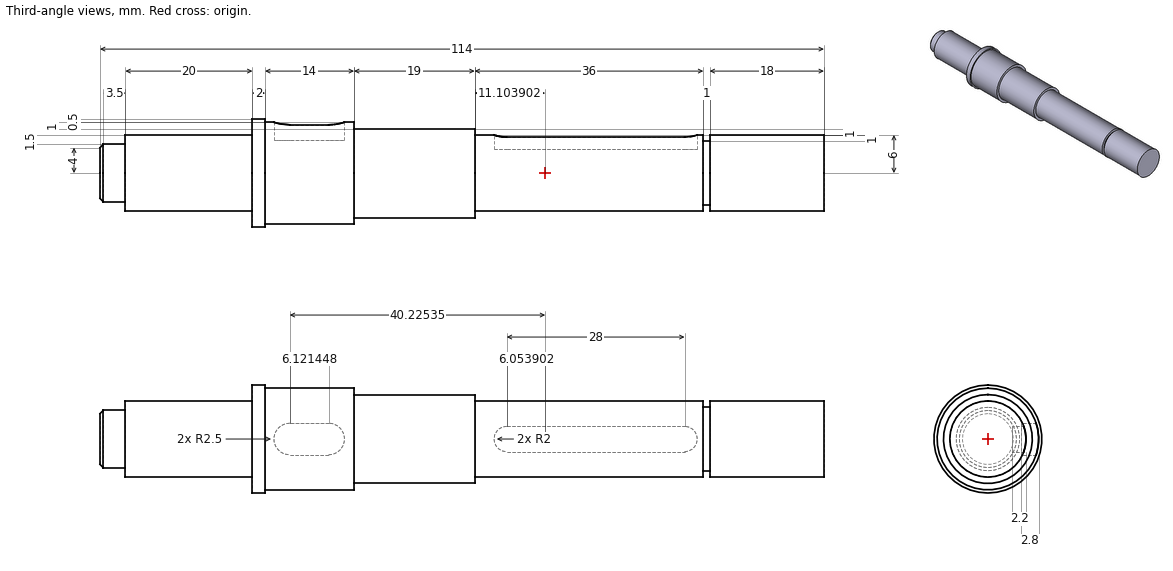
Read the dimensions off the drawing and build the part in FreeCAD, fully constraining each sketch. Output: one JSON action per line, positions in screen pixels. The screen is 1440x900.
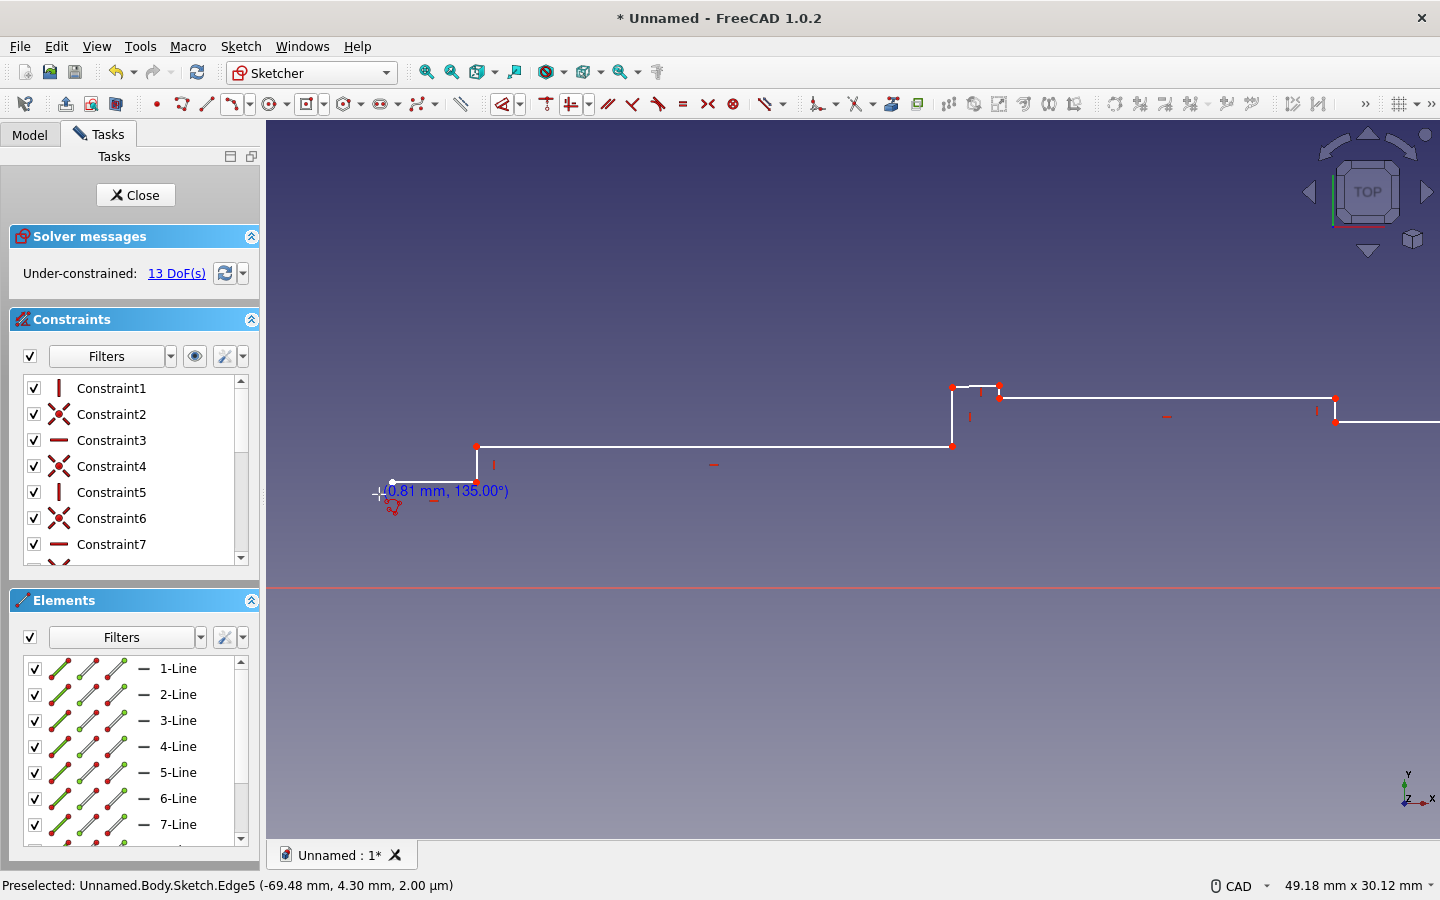
{"action": "left_click", "coordinate": [380, 492]}
{"action": "left_click", "coordinate": [380, 588]}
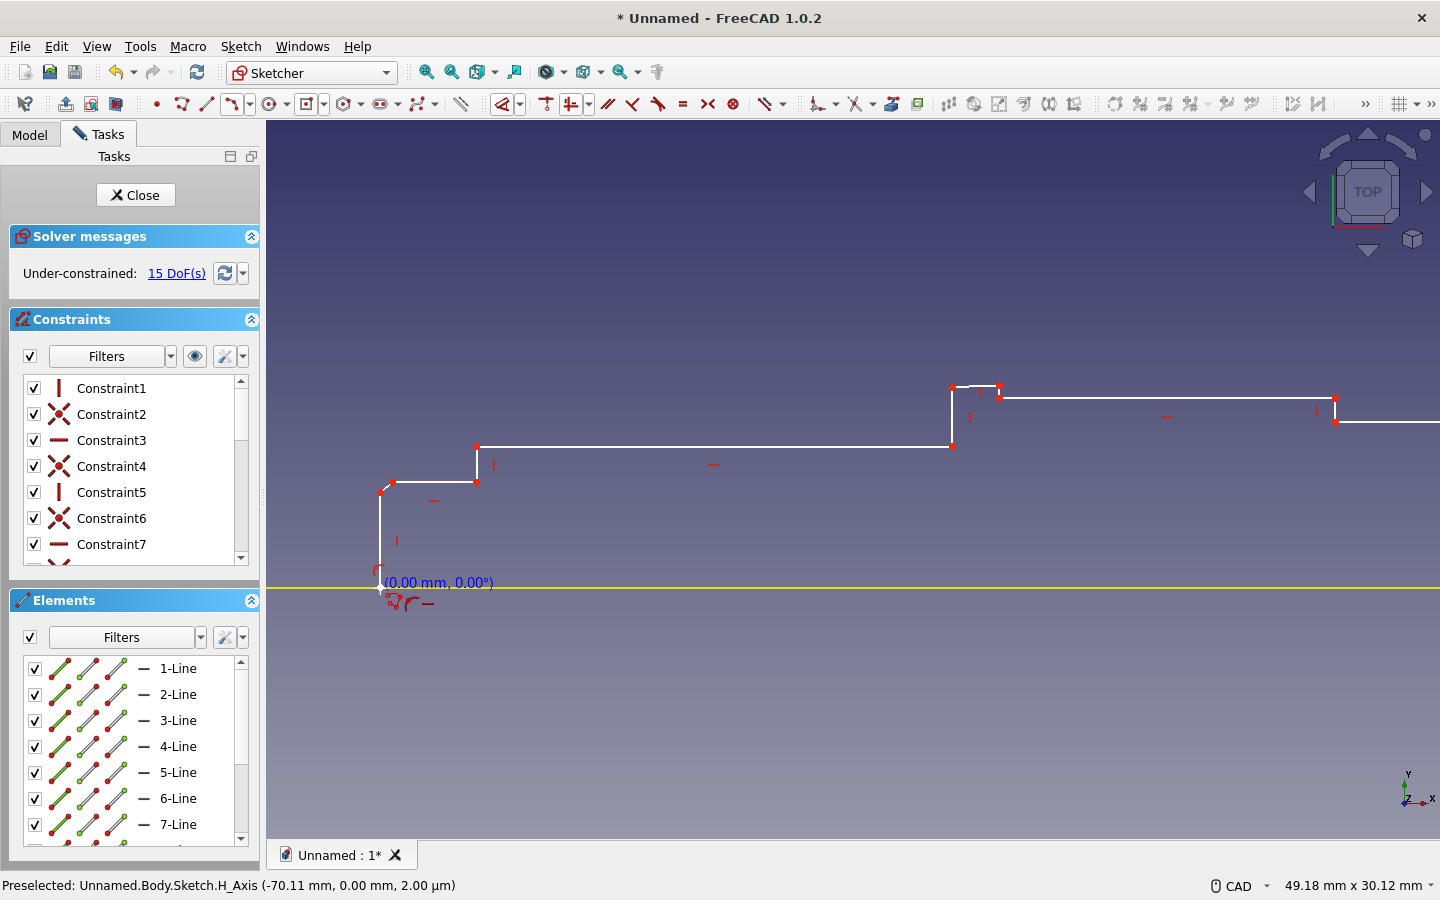
{"action": "scroll", "coordinate": [471, 477], "scroll_direction": "down", "scroll_amount": 7}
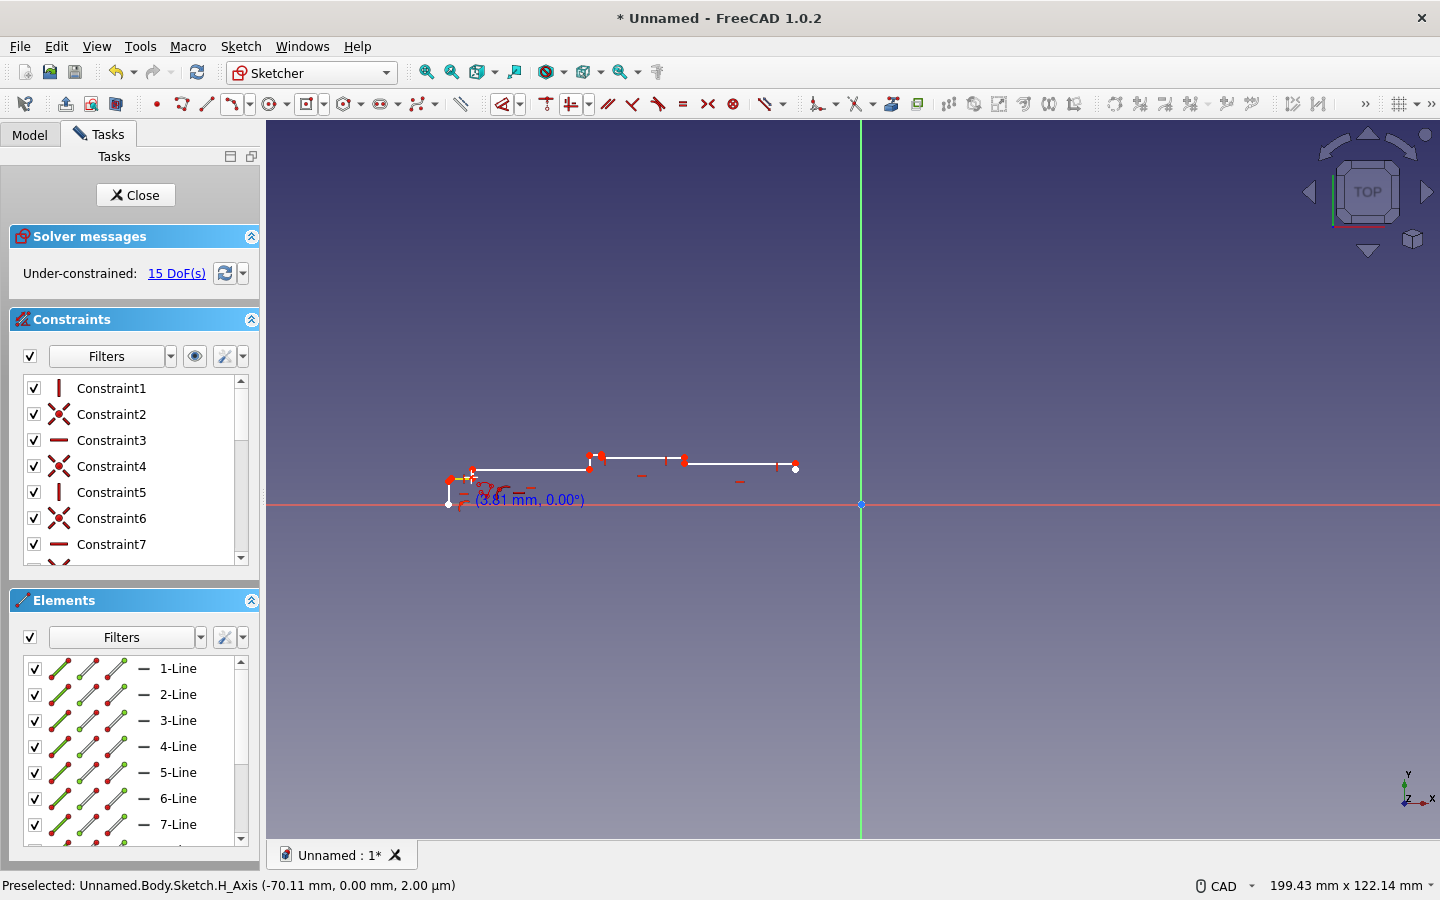
{"action": "left_click", "coordinate": [1120, 496]}
{"action": "left_click", "coordinate": [1120, 469]}
{"action": "left_click", "coordinate": [1014, 469]}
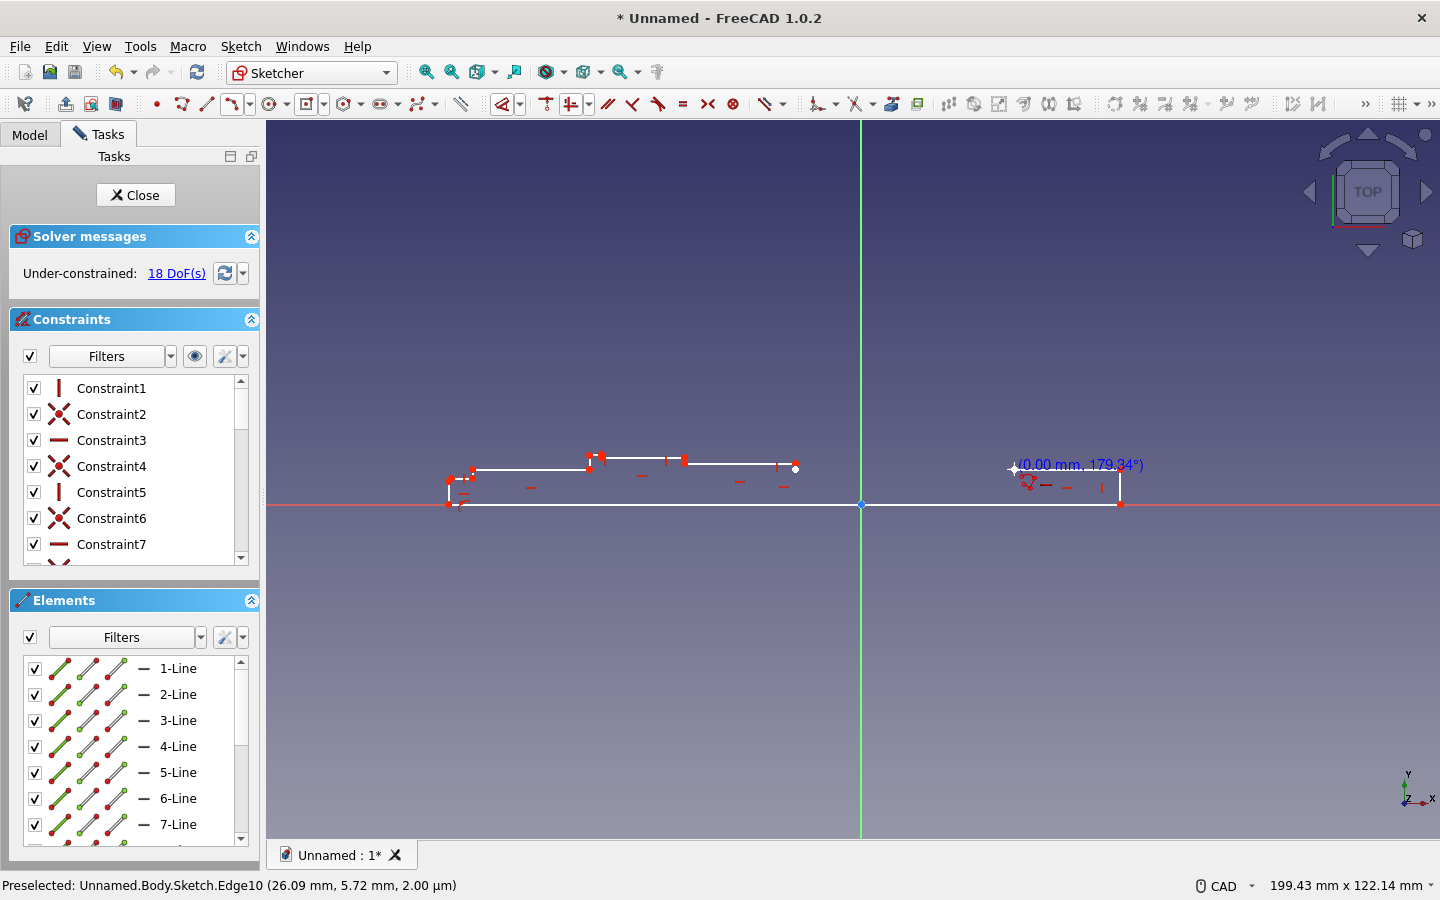
{"action": "scroll", "coordinate": [1014, 475], "scroll_direction": "up", "scroll_amount": 5}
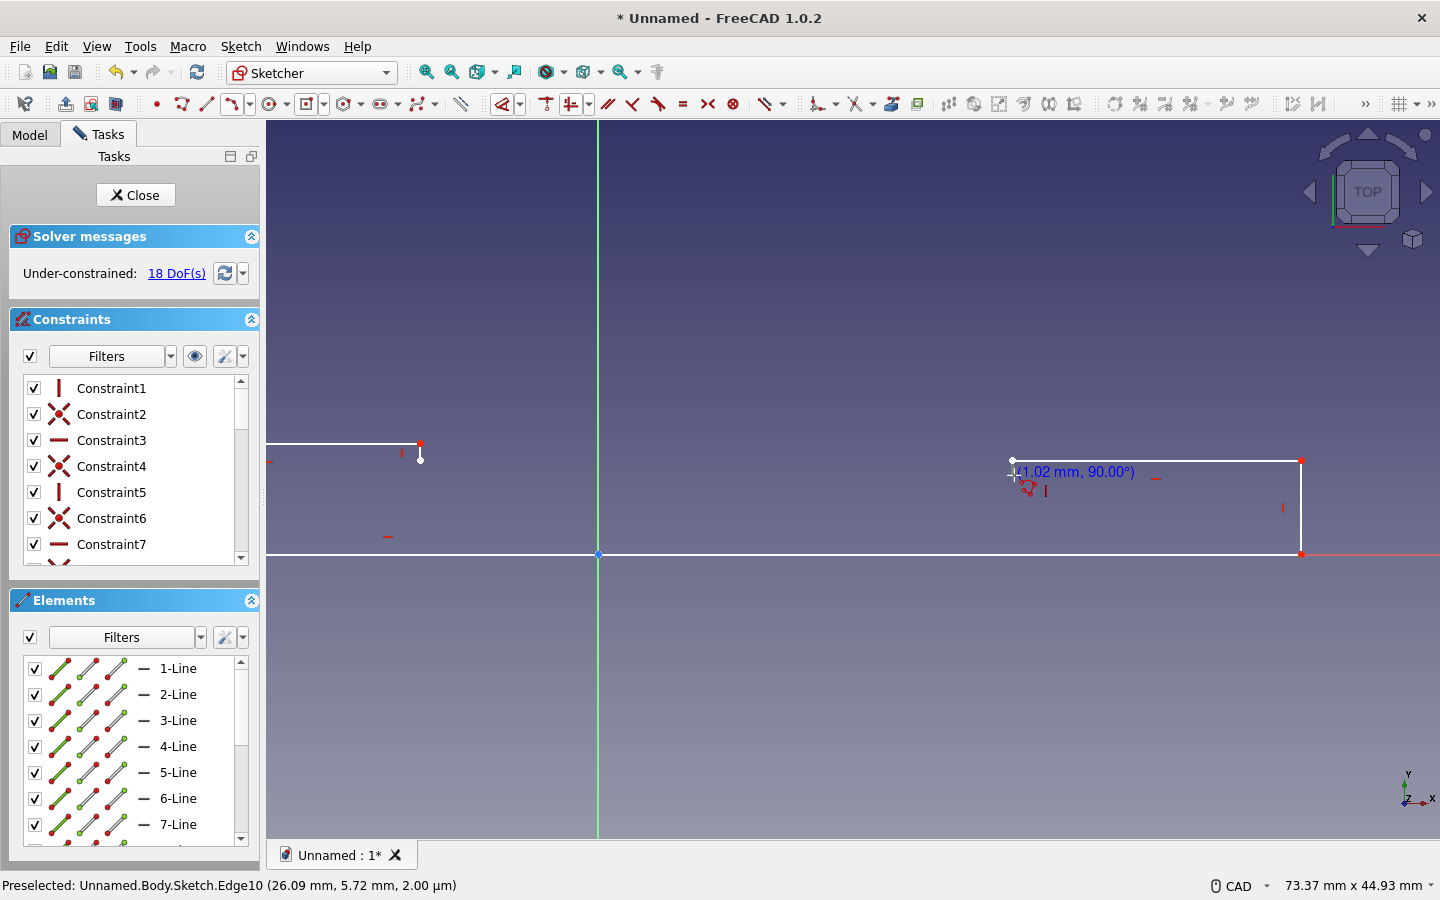
{"action": "left_click", "coordinate": [1013, 475]}
{"action": "left_click", "coordinate": [996, 475]}
{"action": "left_click", "coordinate": [996, 459]}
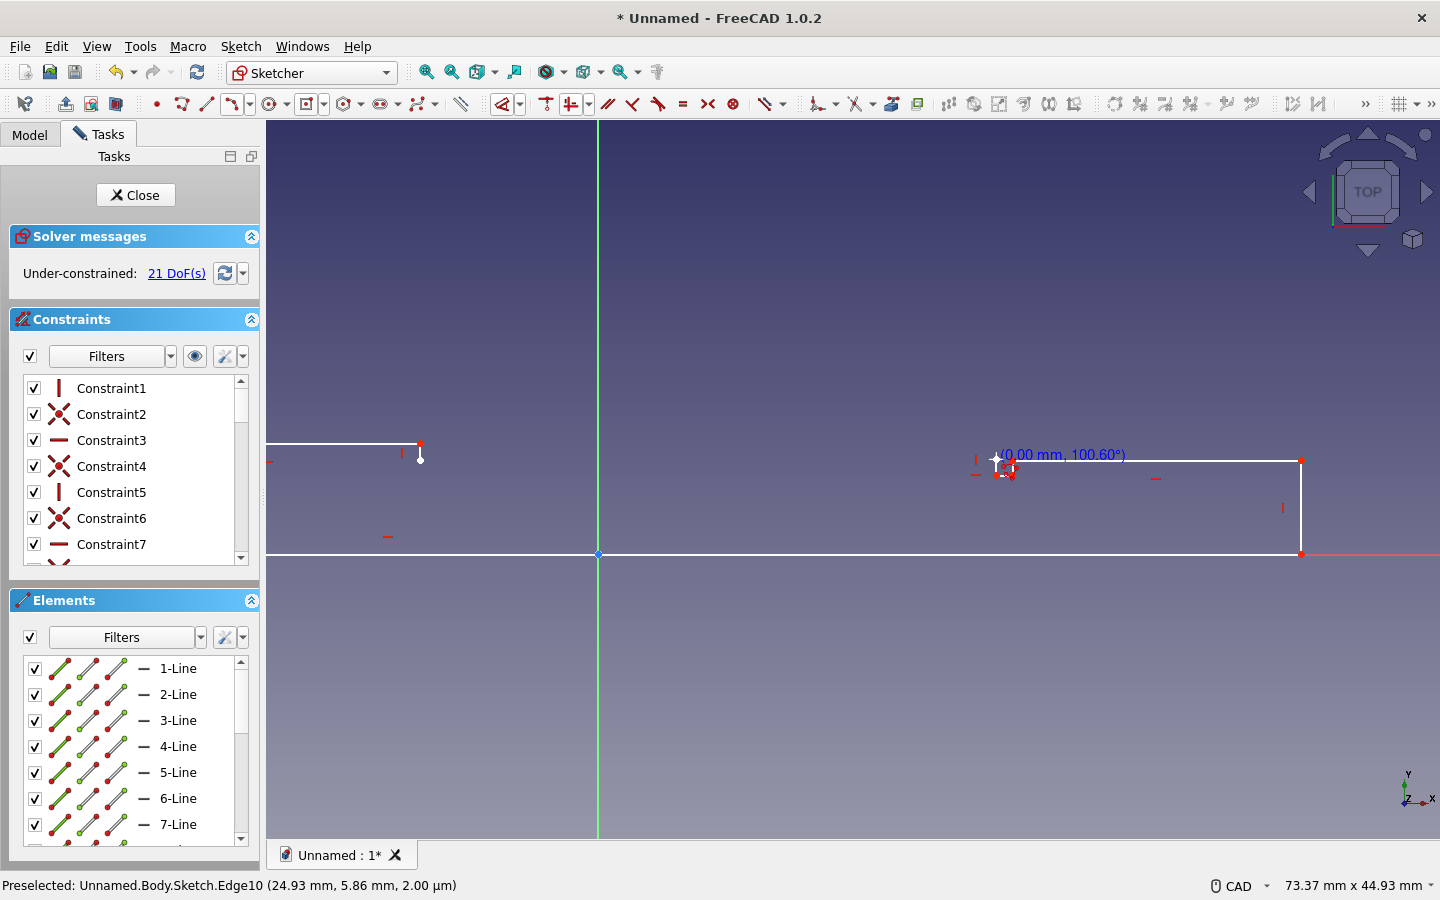
{"action": "scroll", "coordinate": [420, 459], "scroll_direction": "up", "scroll_amount": 4}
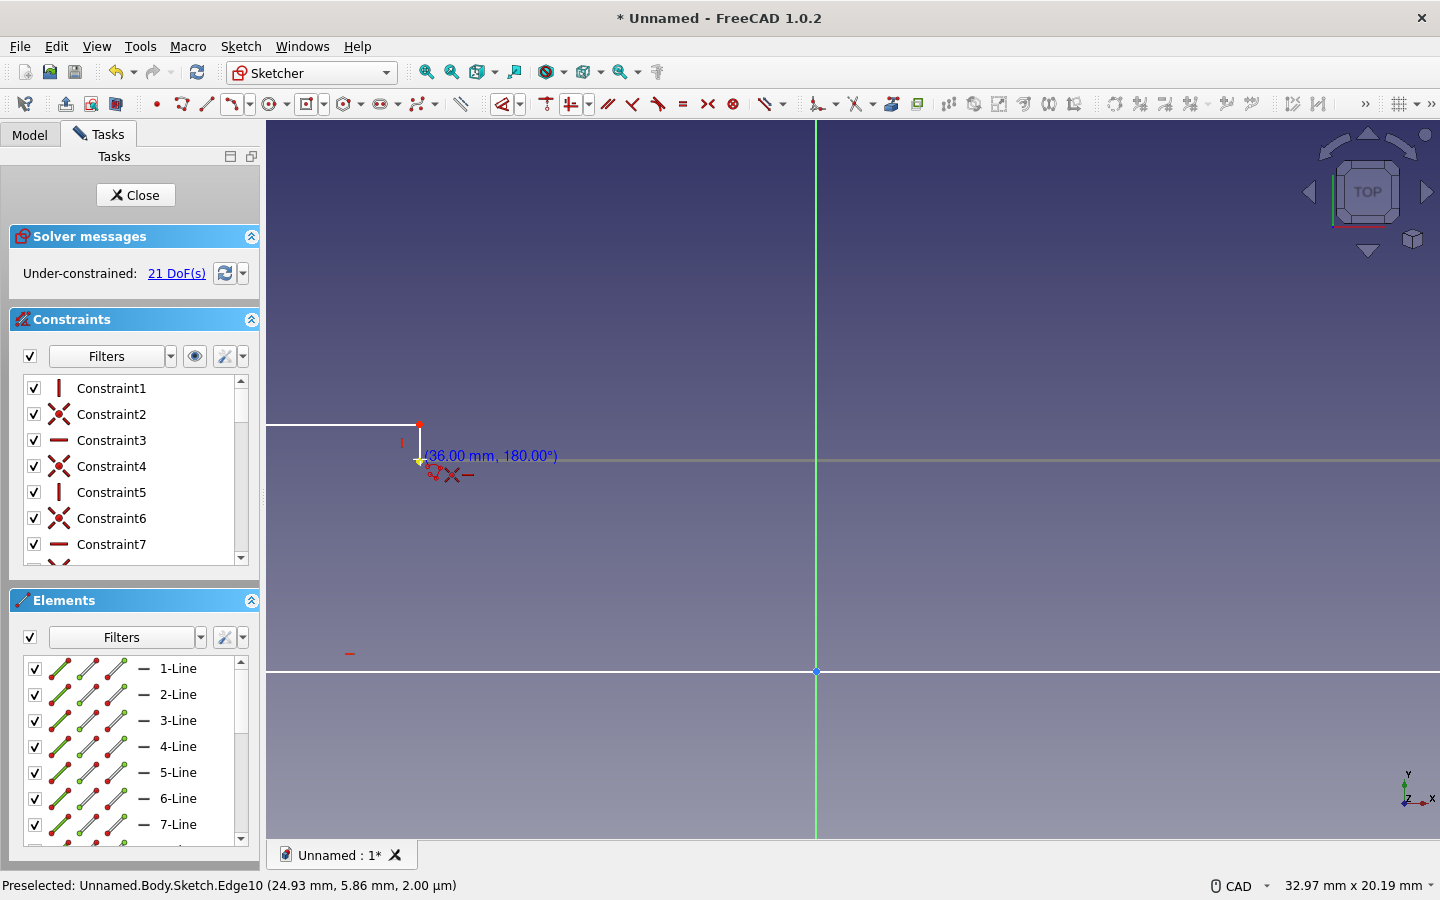
{"action": "left_click", "coordinate": [420, 461]}
{"action": "key", "text": "Escape"}
{"action": "key", "text": "Escape"}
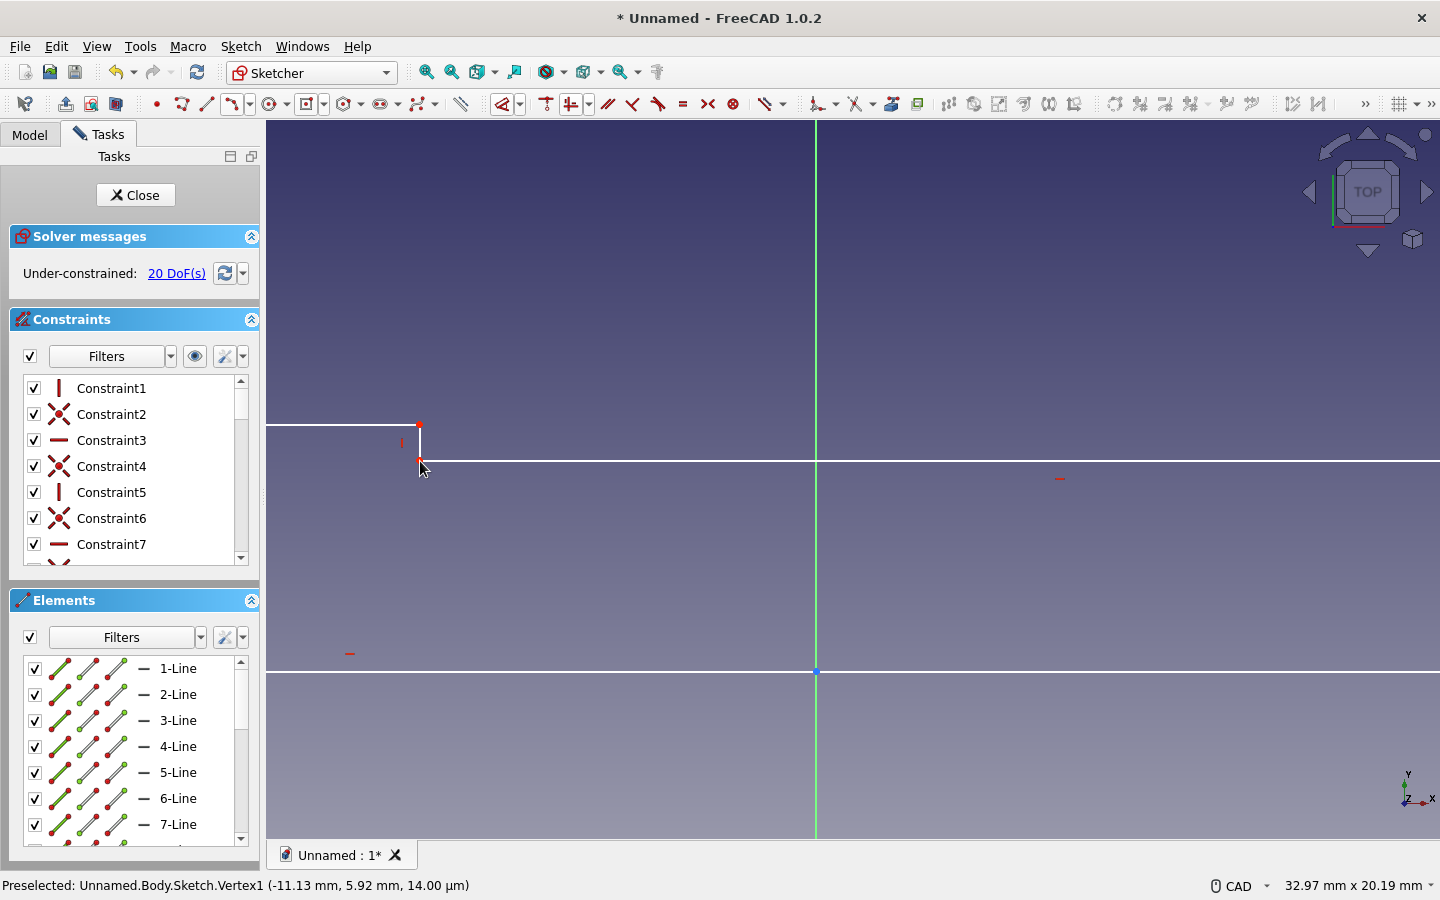
{"action": "scroll", "coordinate": [871, 471], "scroll_direction": "down", "scroll_amount": 9}